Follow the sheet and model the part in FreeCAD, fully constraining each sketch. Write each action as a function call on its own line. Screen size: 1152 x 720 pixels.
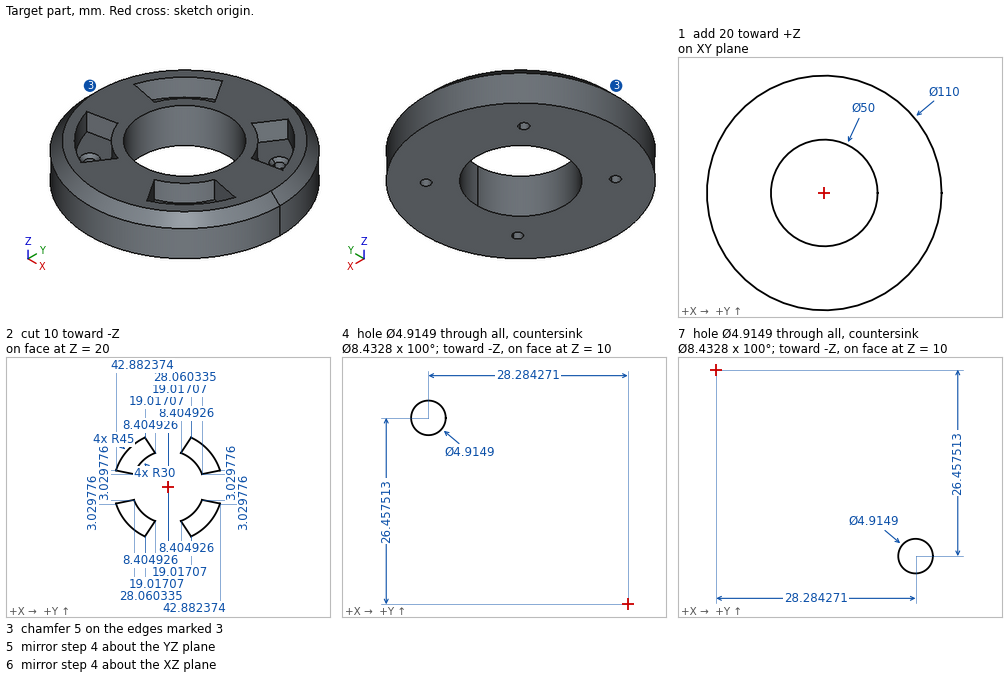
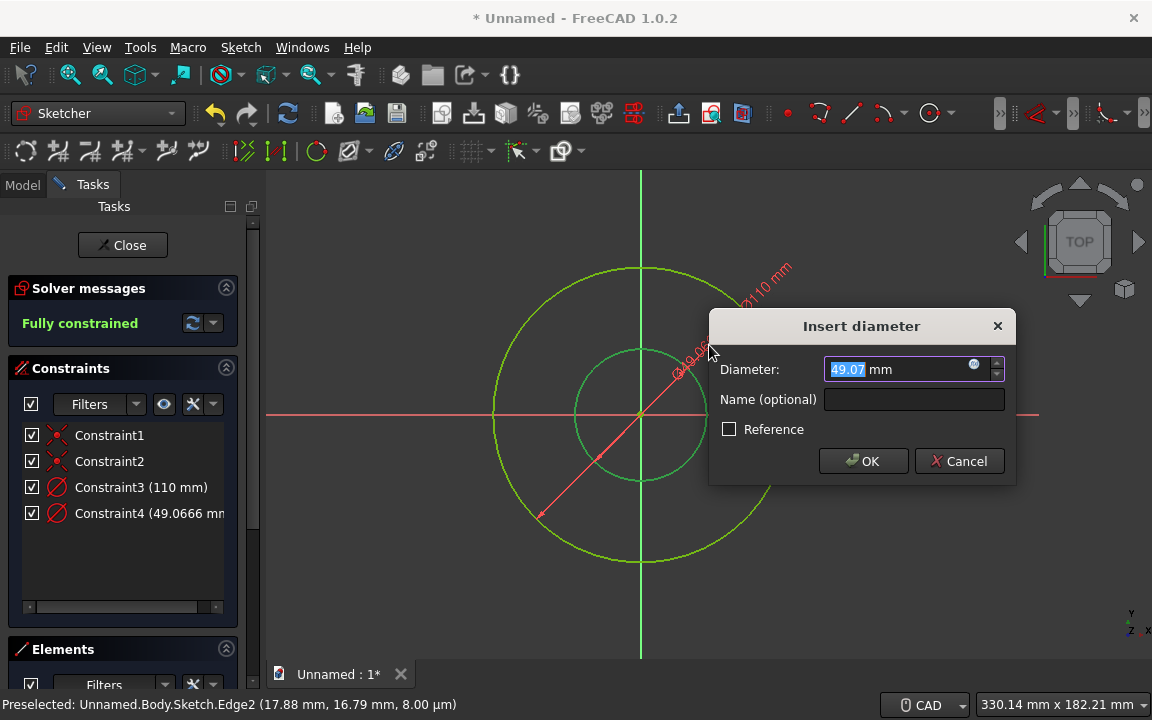
text(50)
key(Return)
key(Escape)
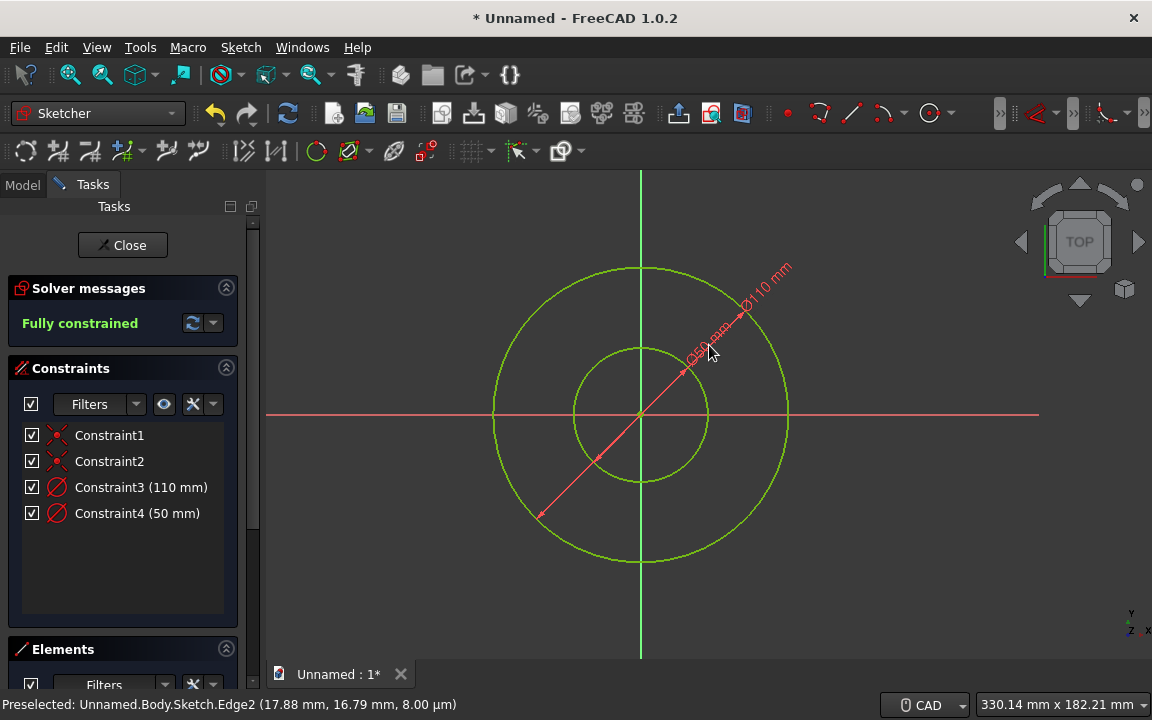
click(123, 245)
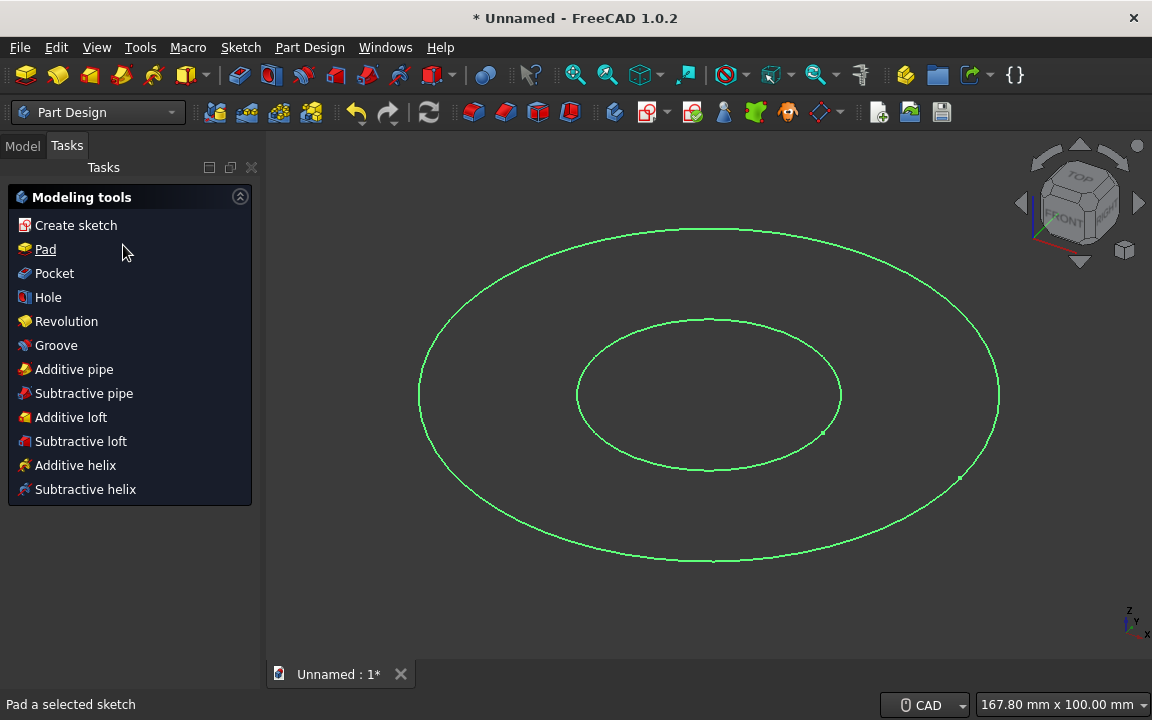
click(26, 76)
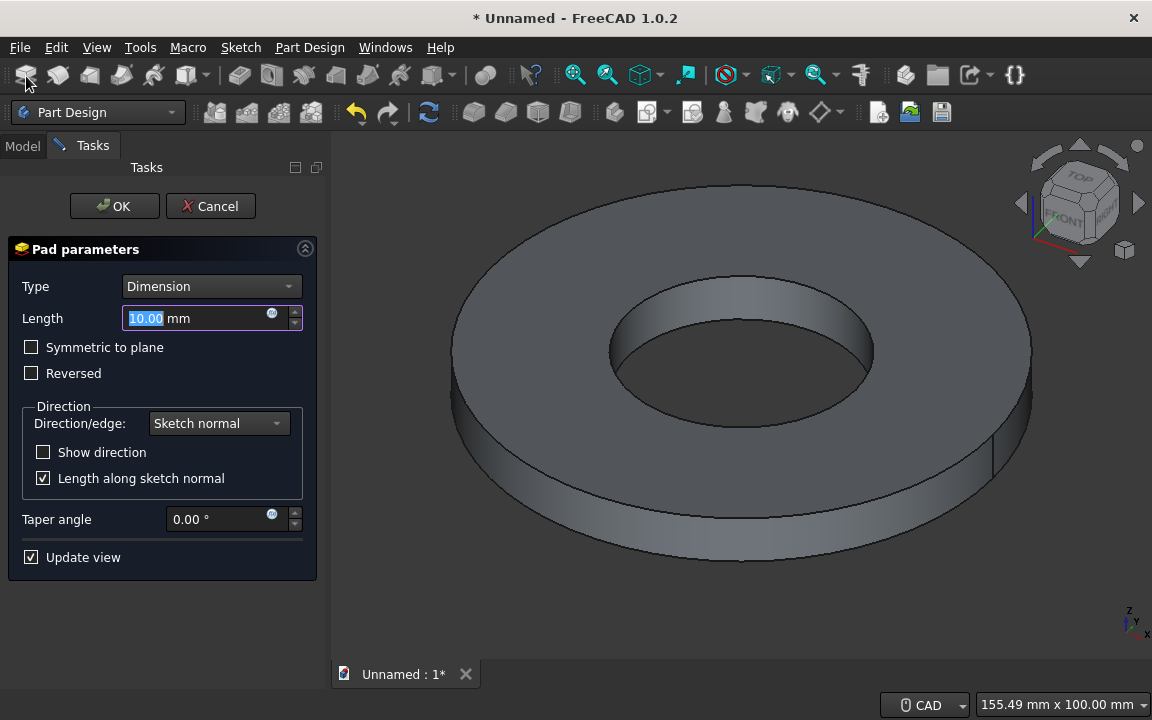
text(20)
key(Tab)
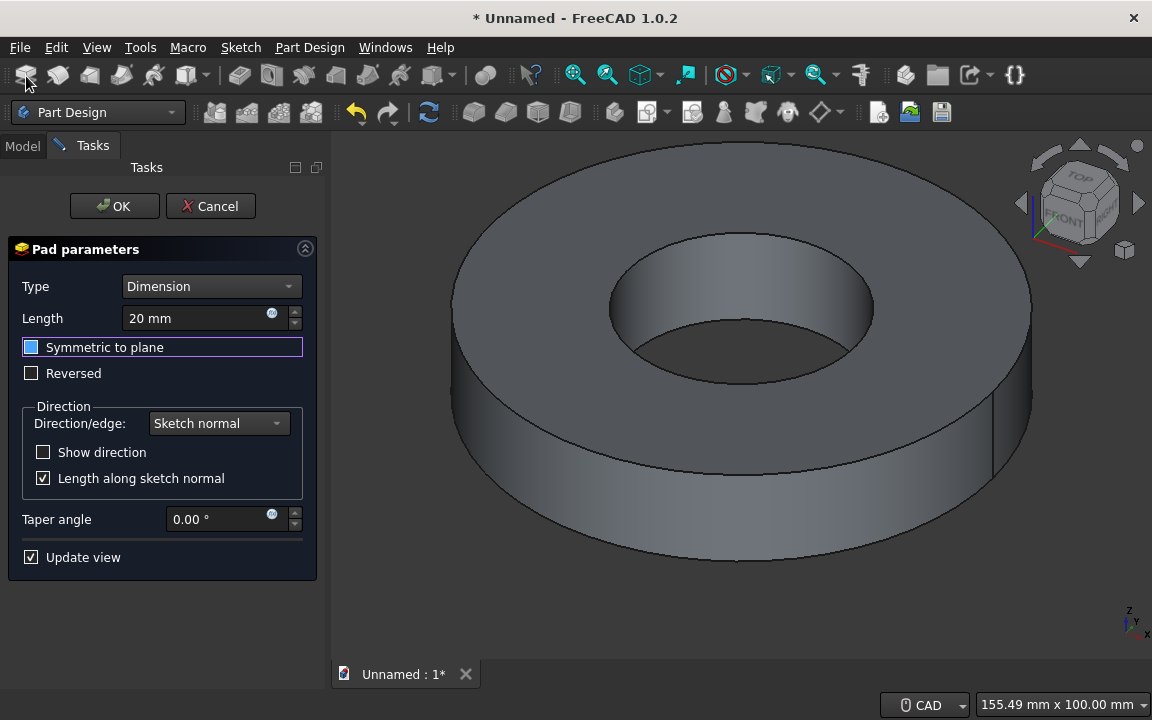
click(115, 206)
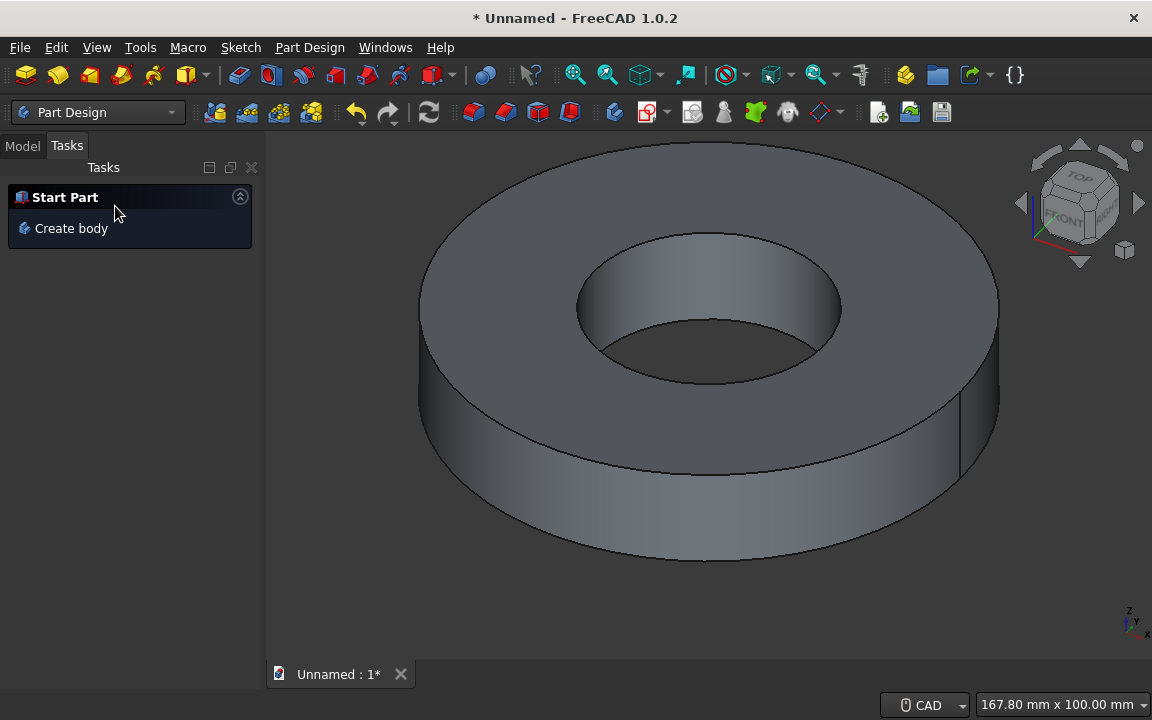
click(576, 76)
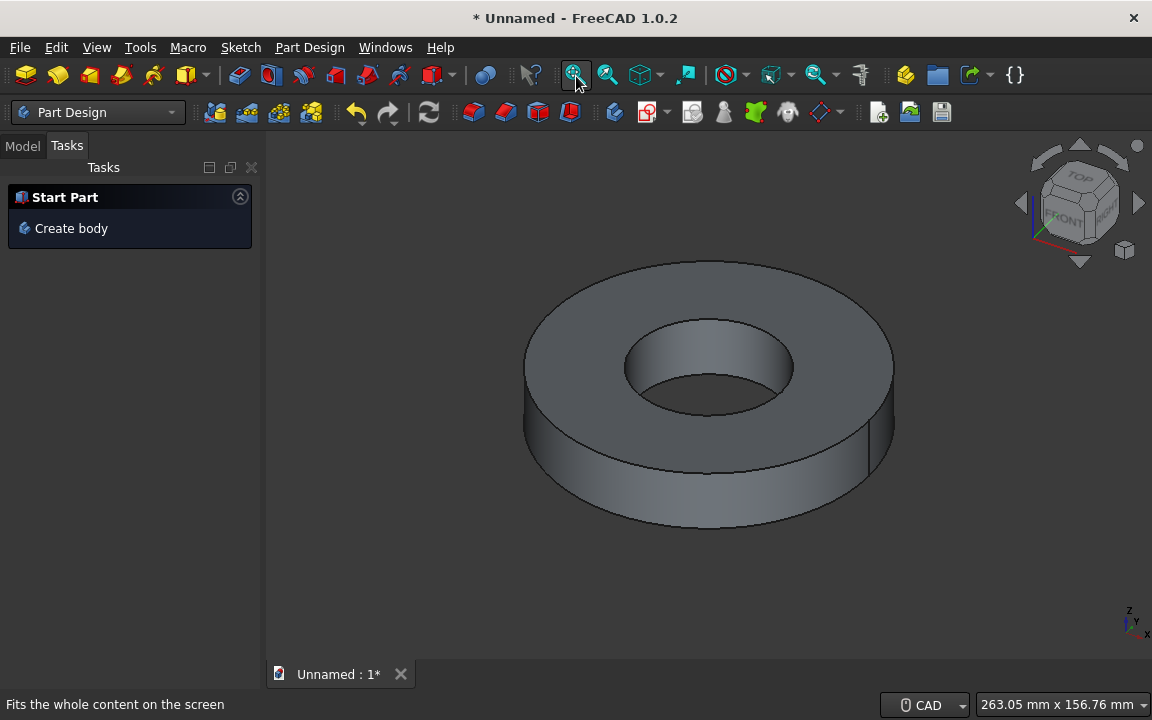
click(564, 389)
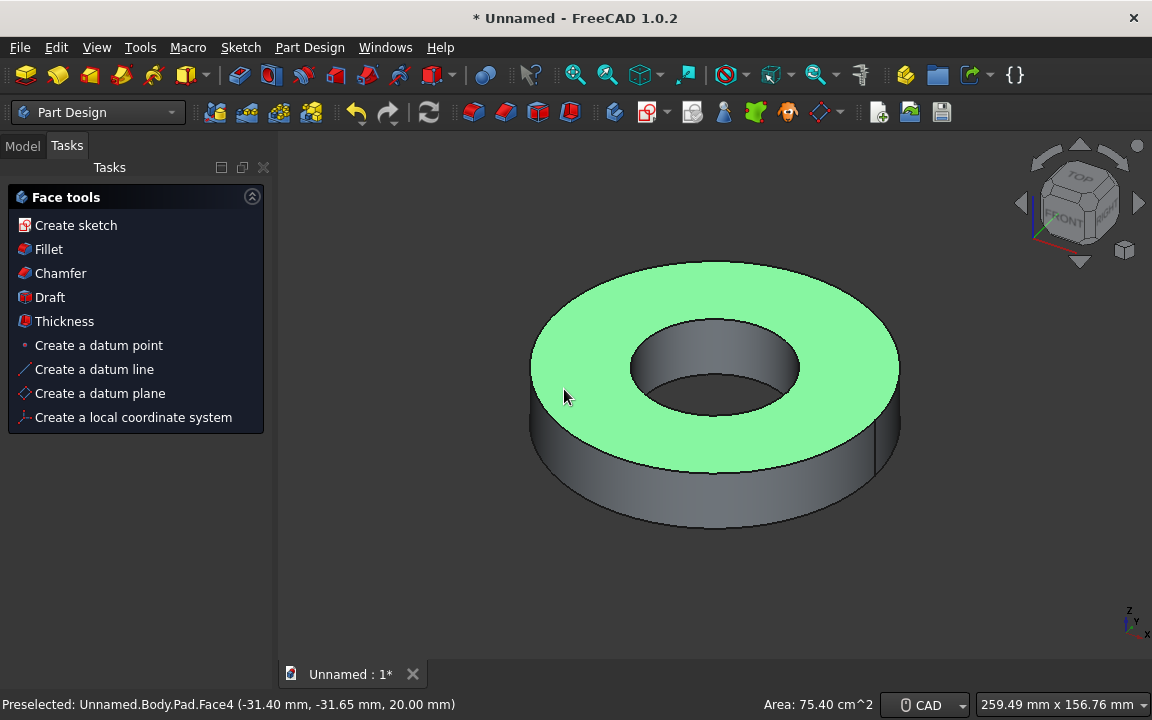
click(648, 112)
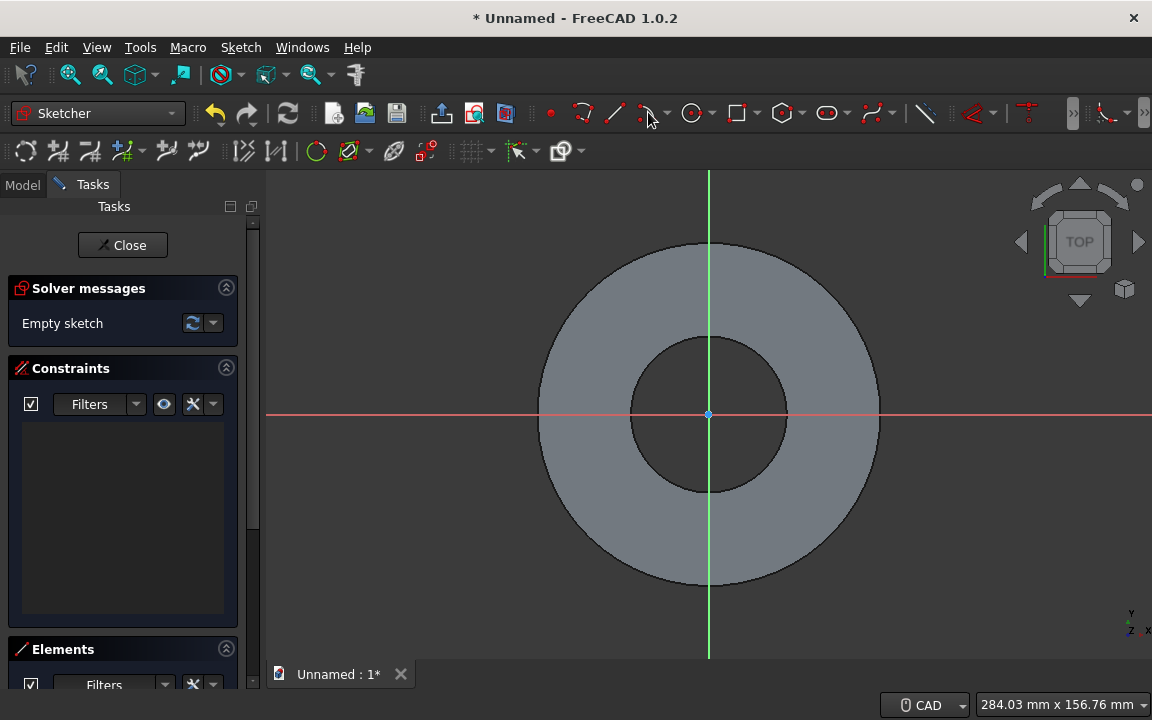
click(616, 114)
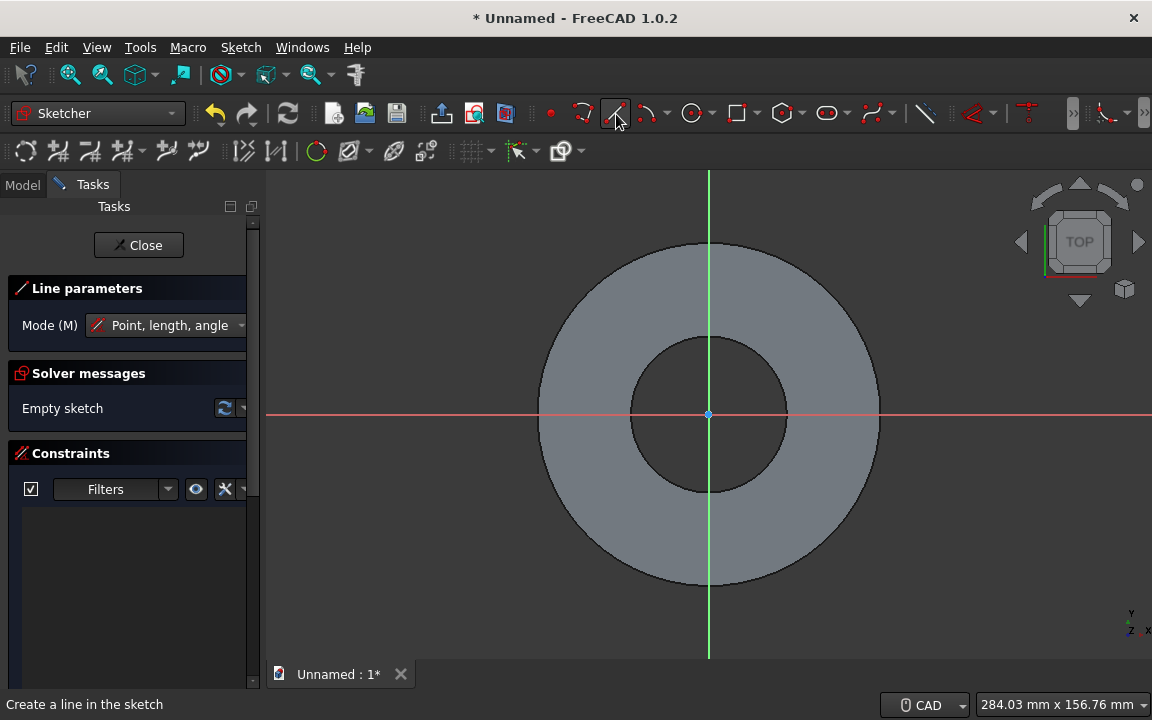
click(676, 327)
click(650, 287)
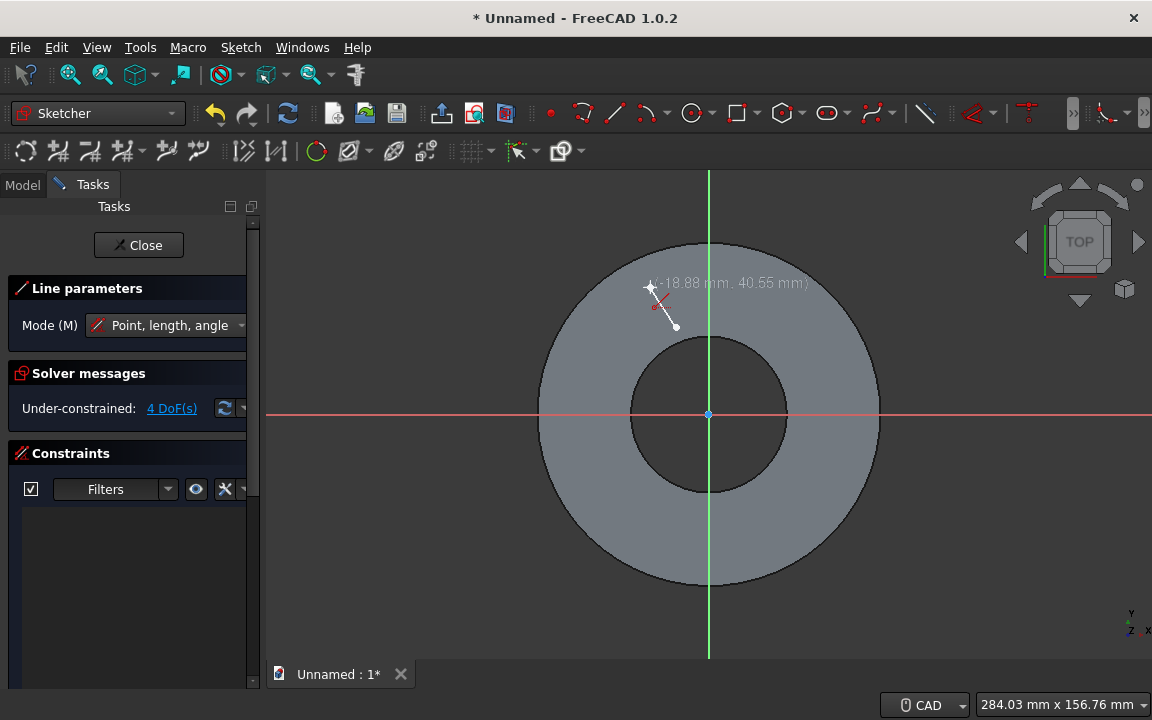
click(575, 372)
click(621, 381)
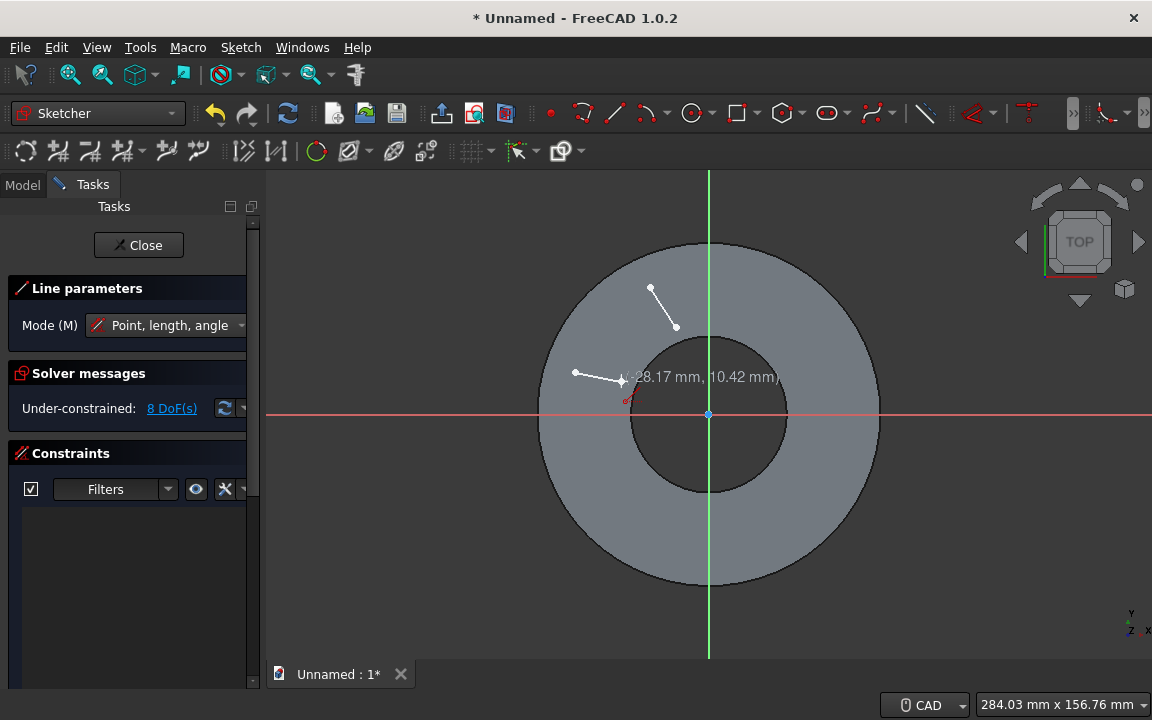
click(670, 114)